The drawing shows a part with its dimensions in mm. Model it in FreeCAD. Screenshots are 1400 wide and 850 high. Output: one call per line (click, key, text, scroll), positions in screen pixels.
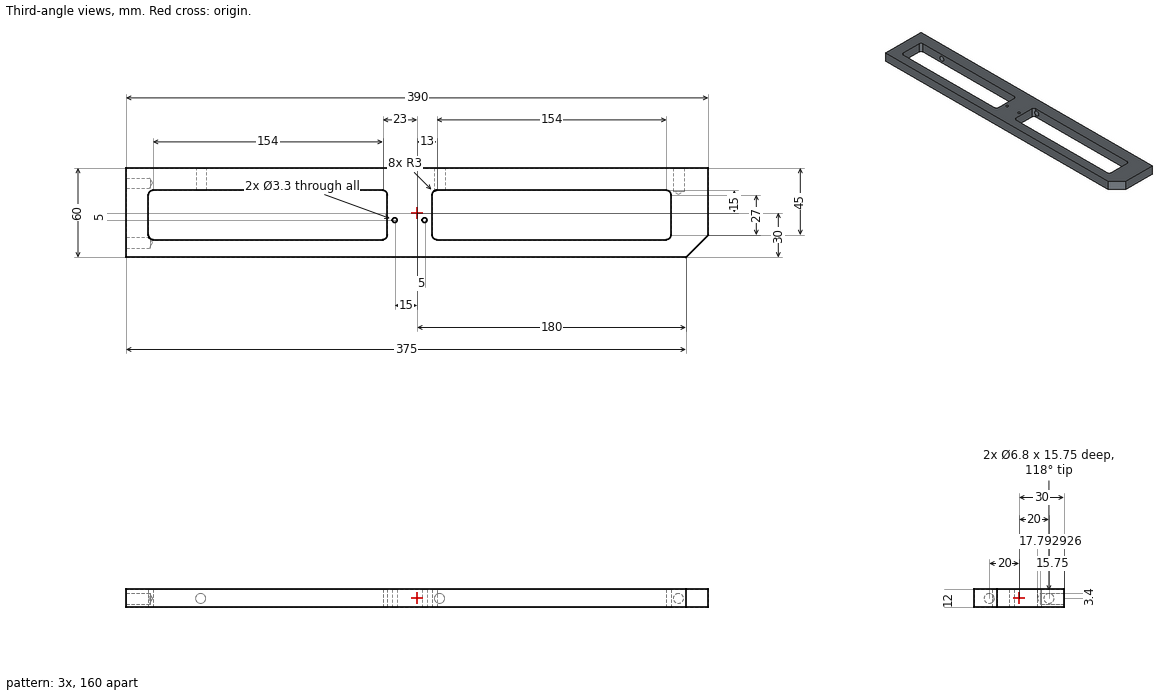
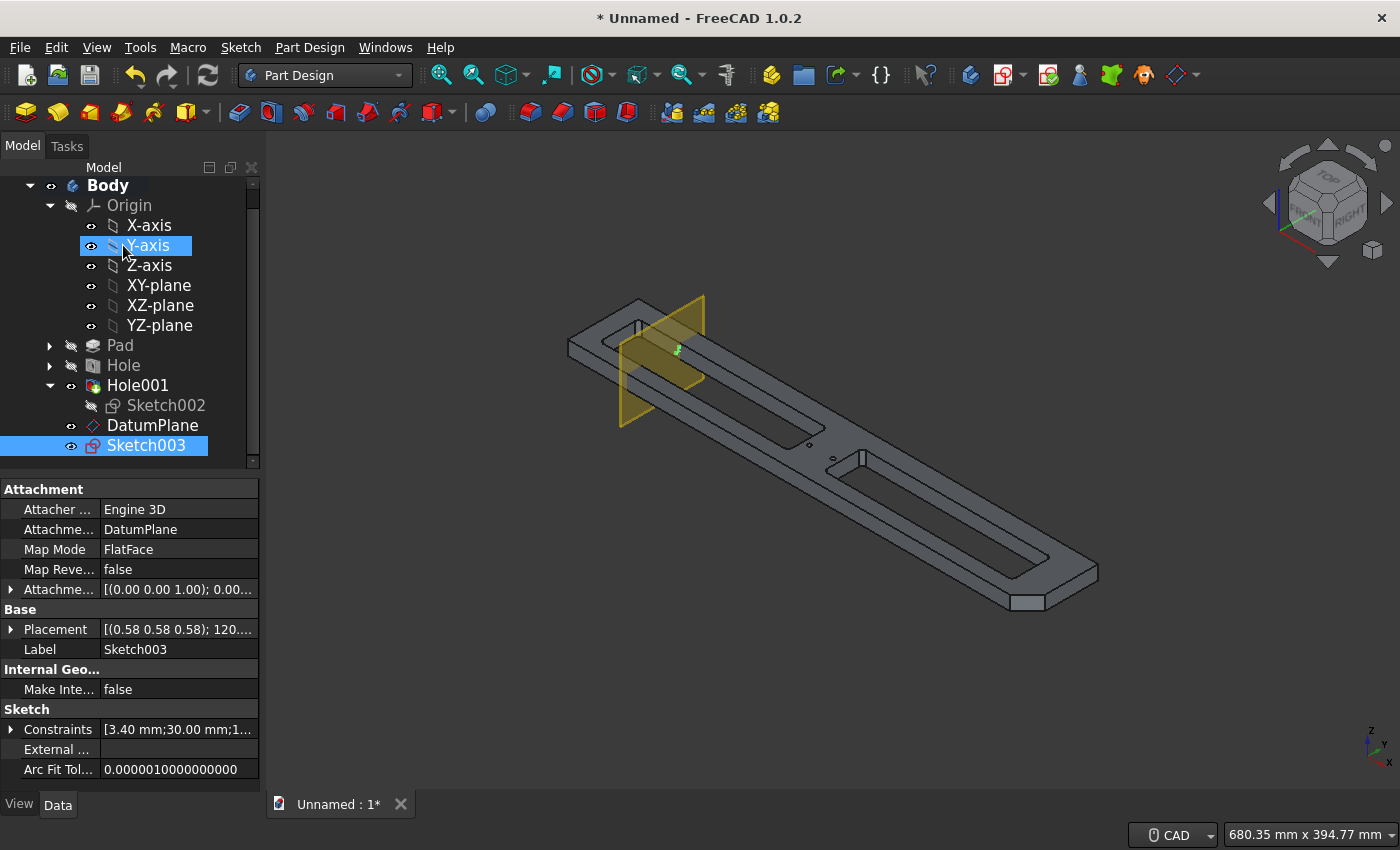
click(304, 112)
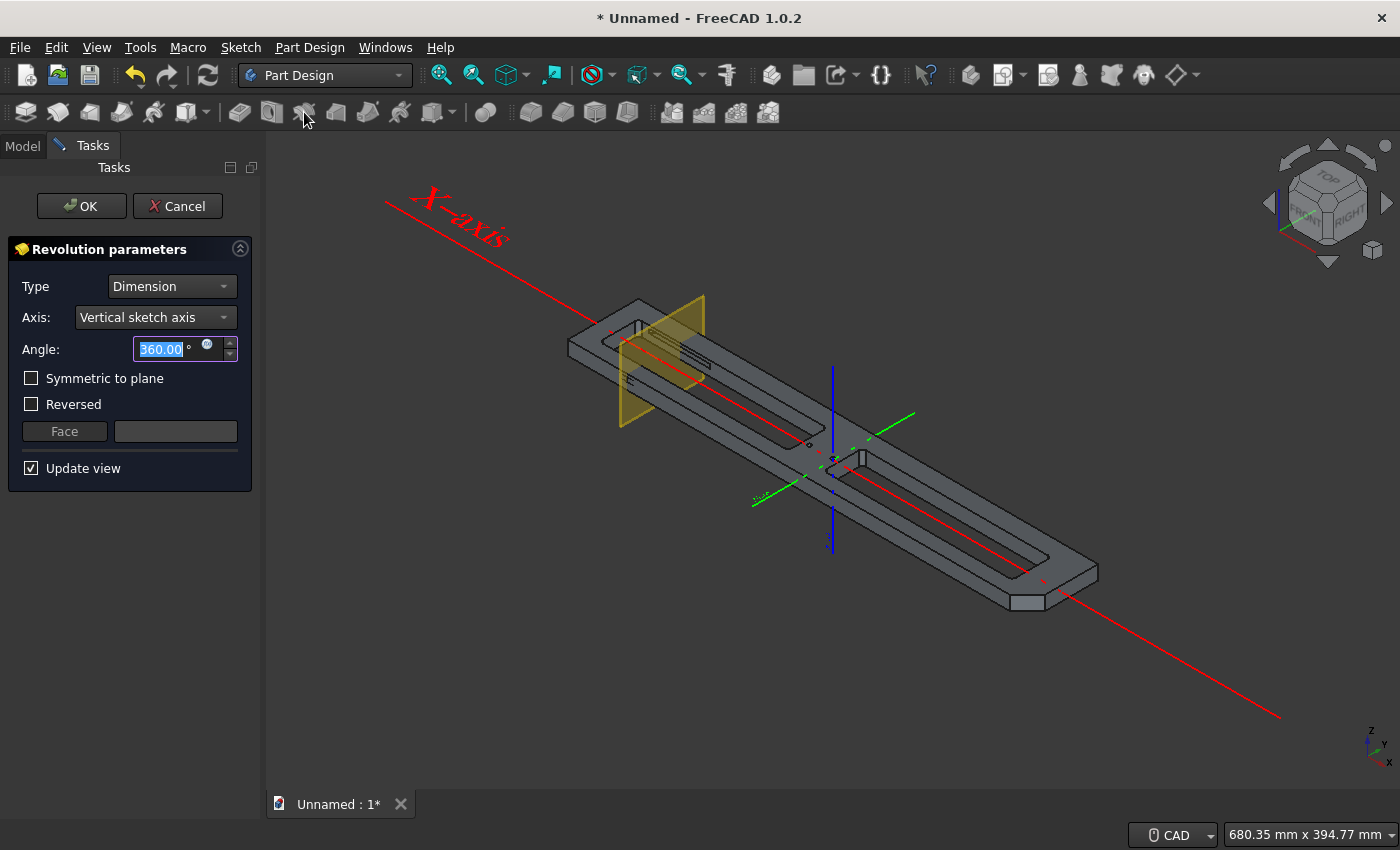
click(156, 318)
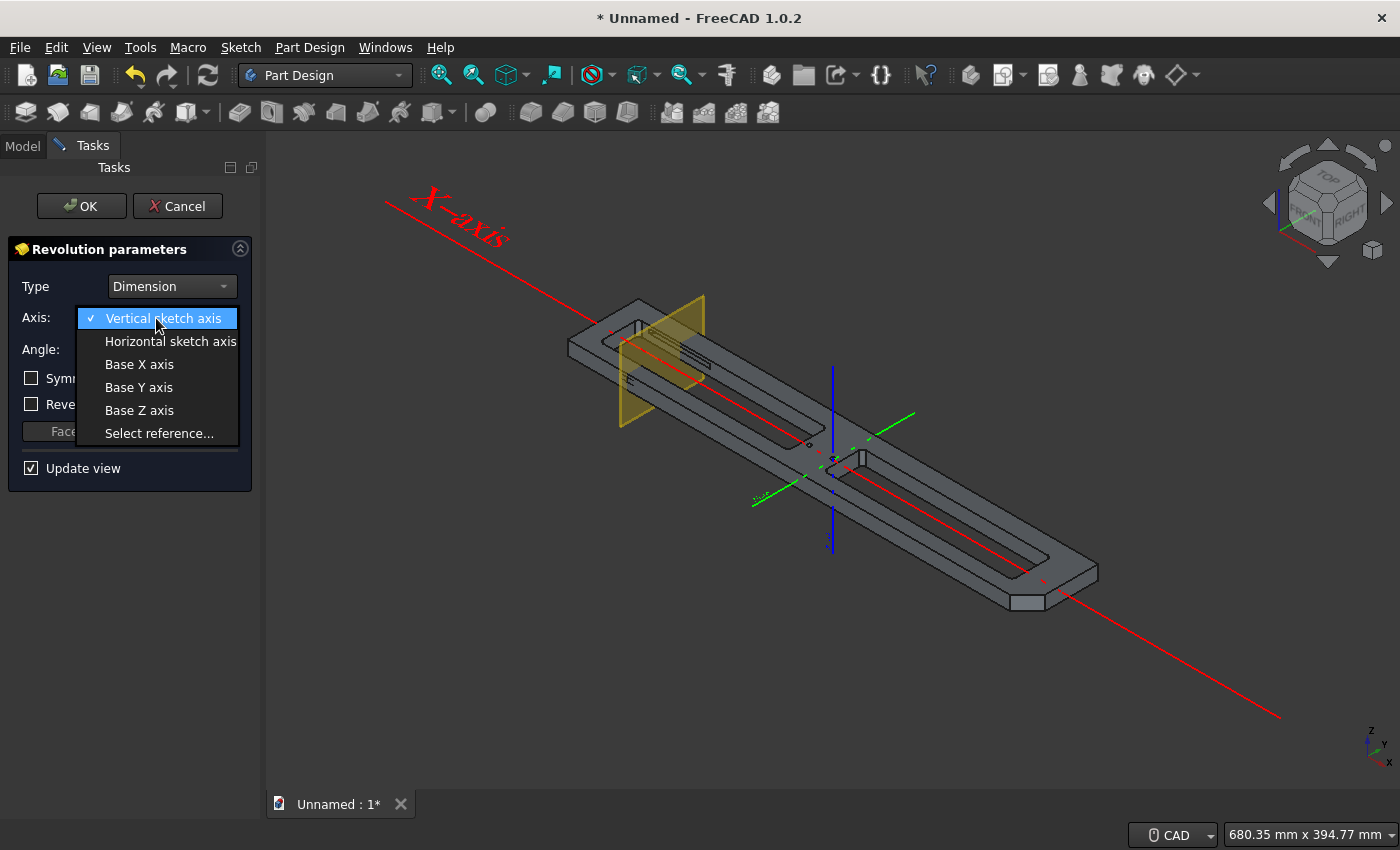
click(156, 342)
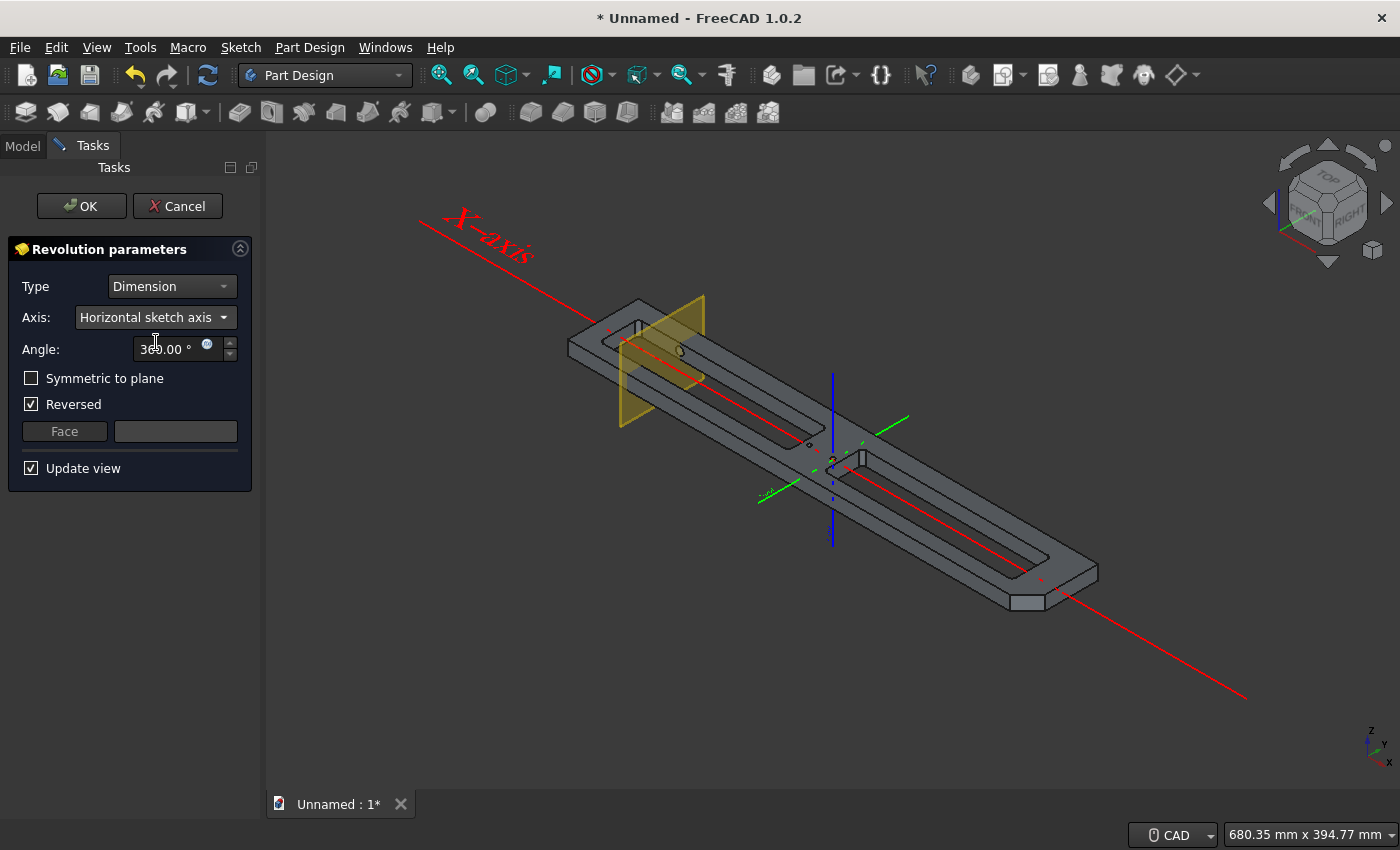
click(82, 206)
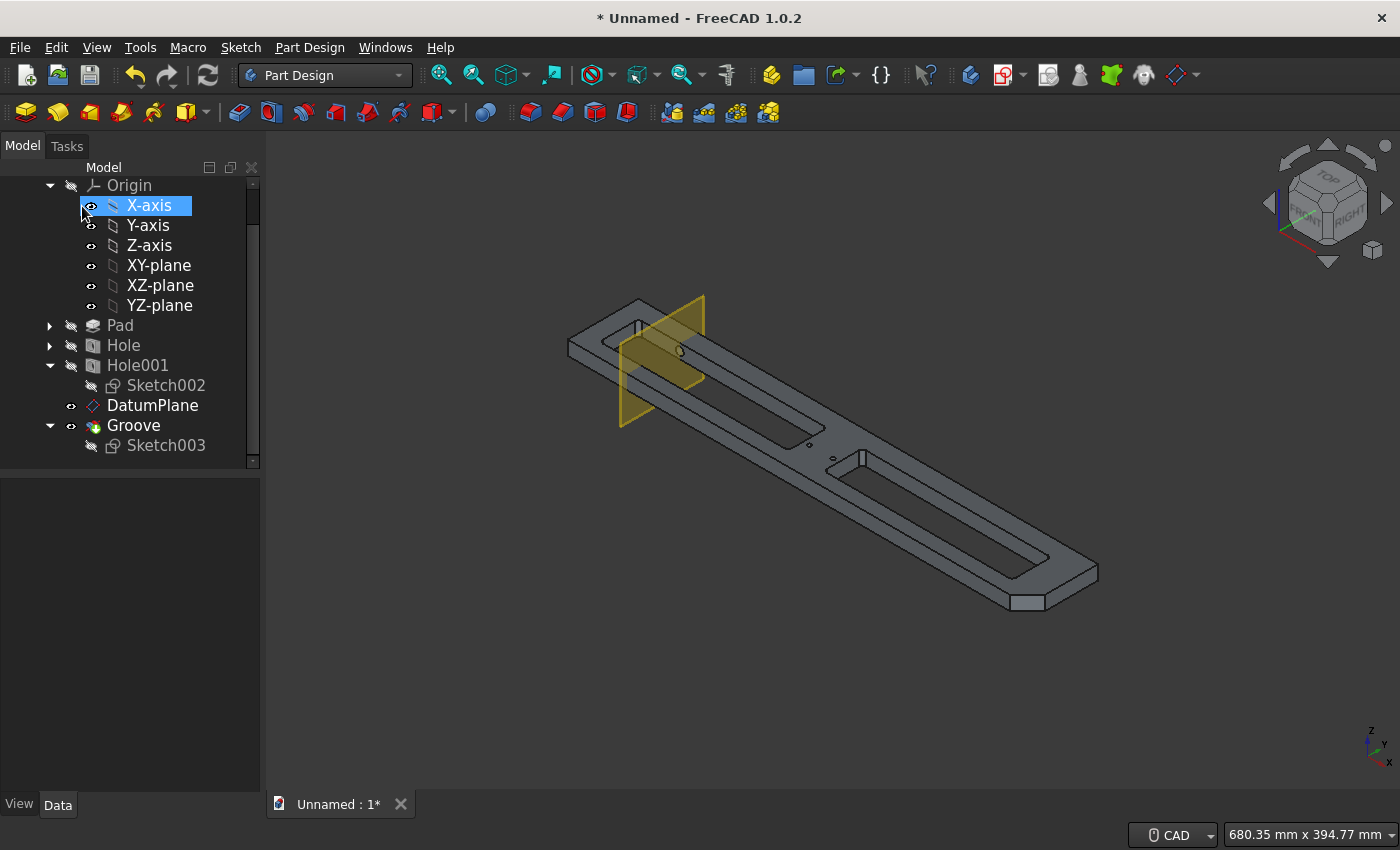
click(116, 406)
key(space)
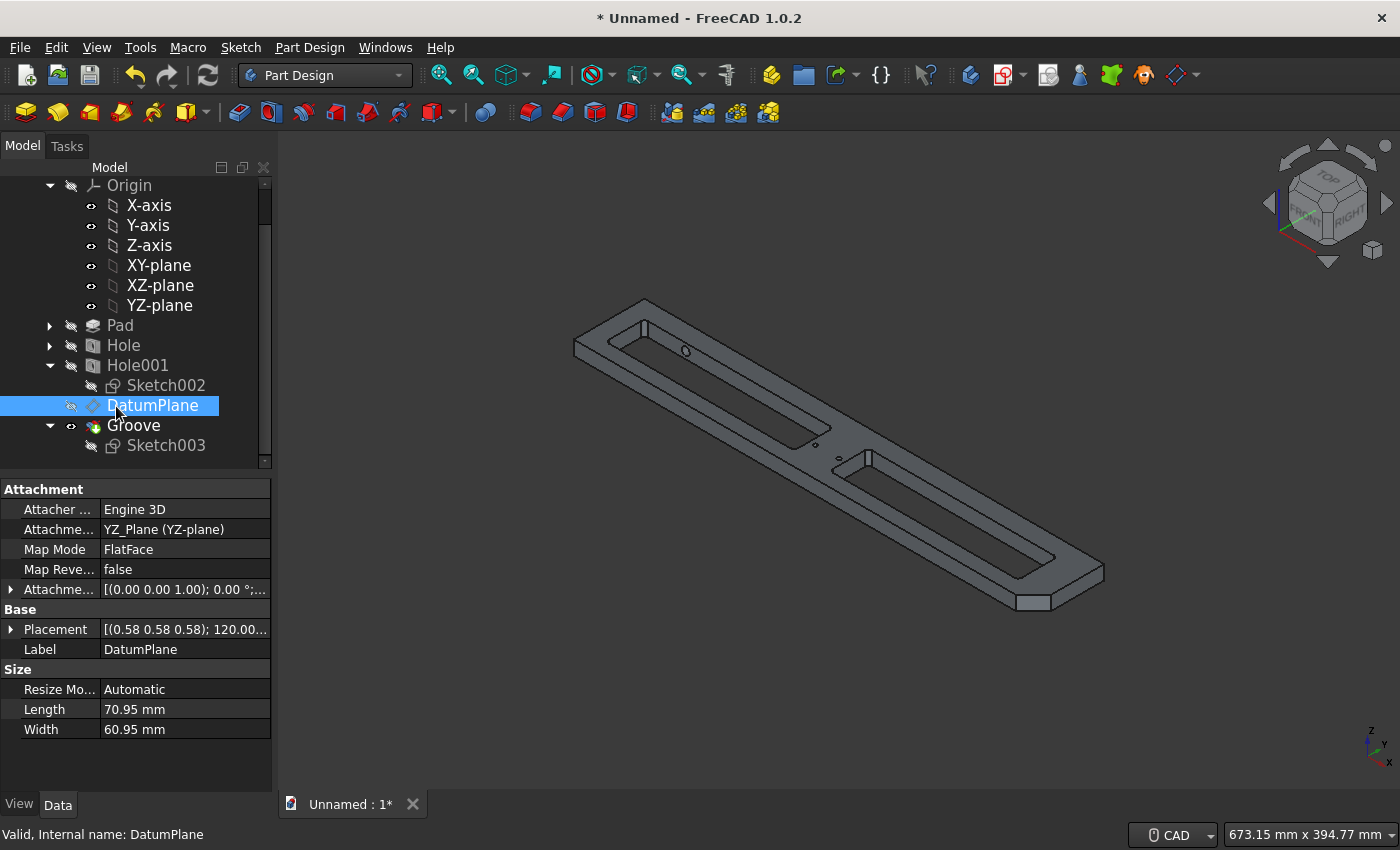
click(116, 426)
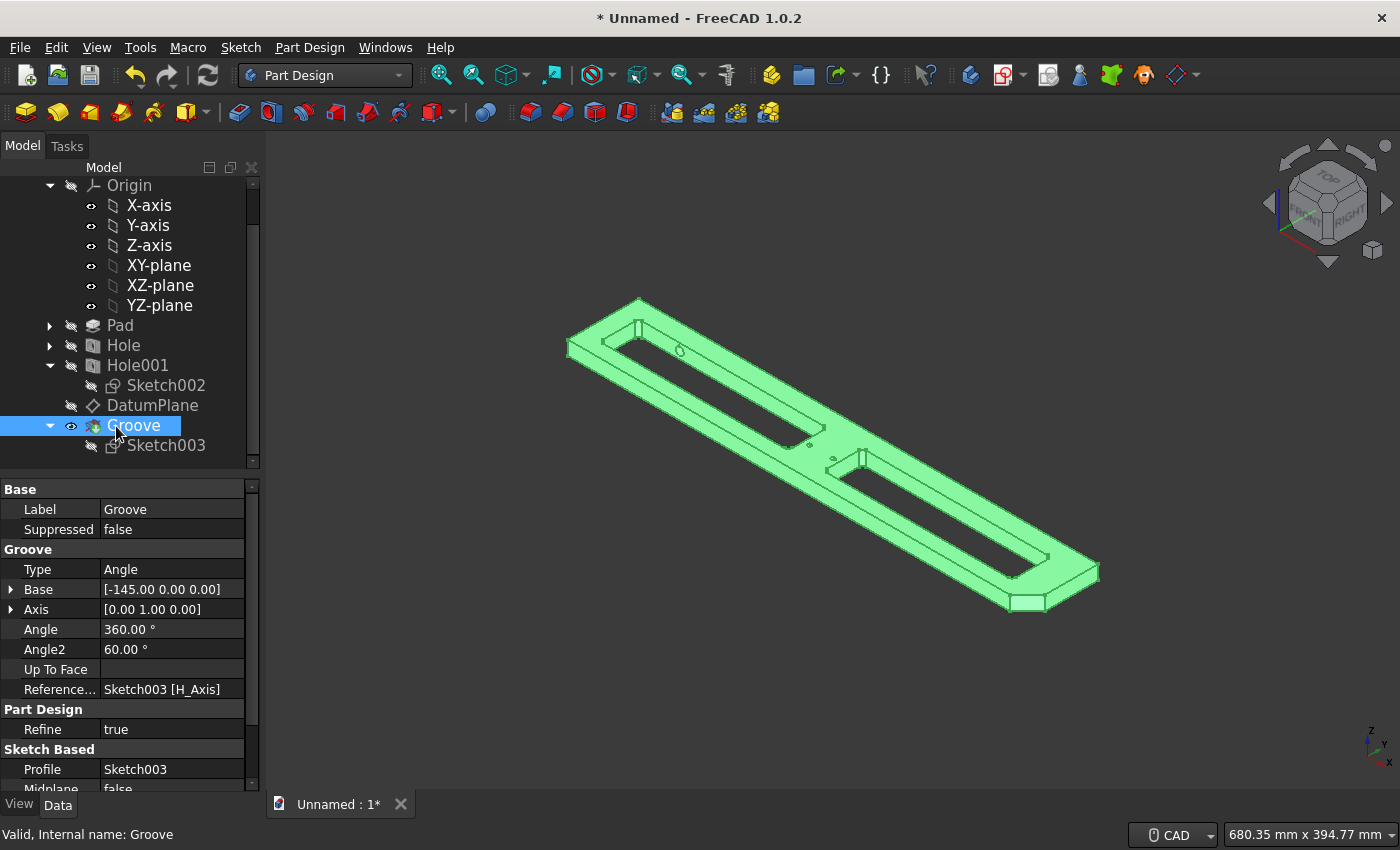
click(704, 112)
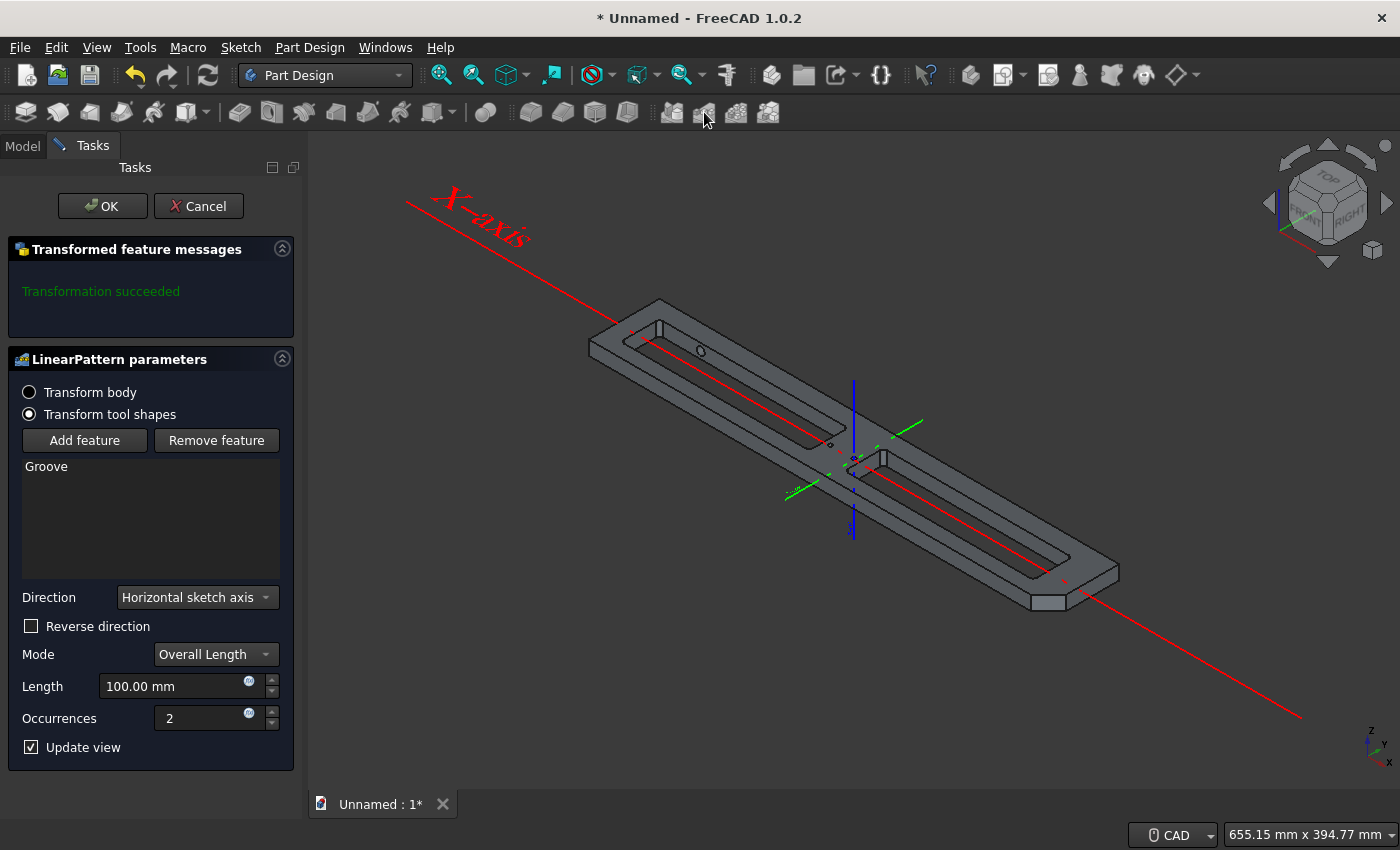
click(198, 598)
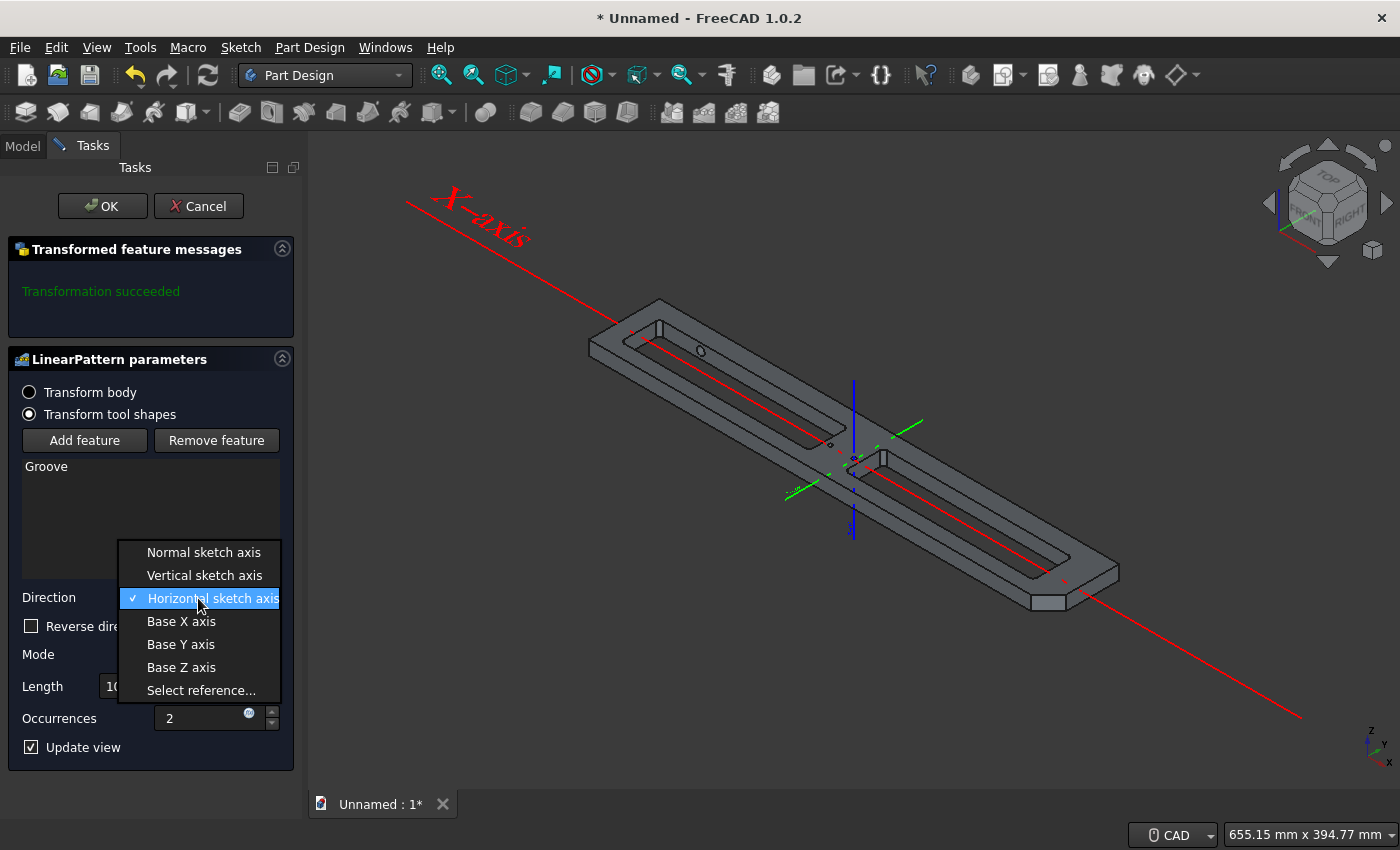
click(198, 622)